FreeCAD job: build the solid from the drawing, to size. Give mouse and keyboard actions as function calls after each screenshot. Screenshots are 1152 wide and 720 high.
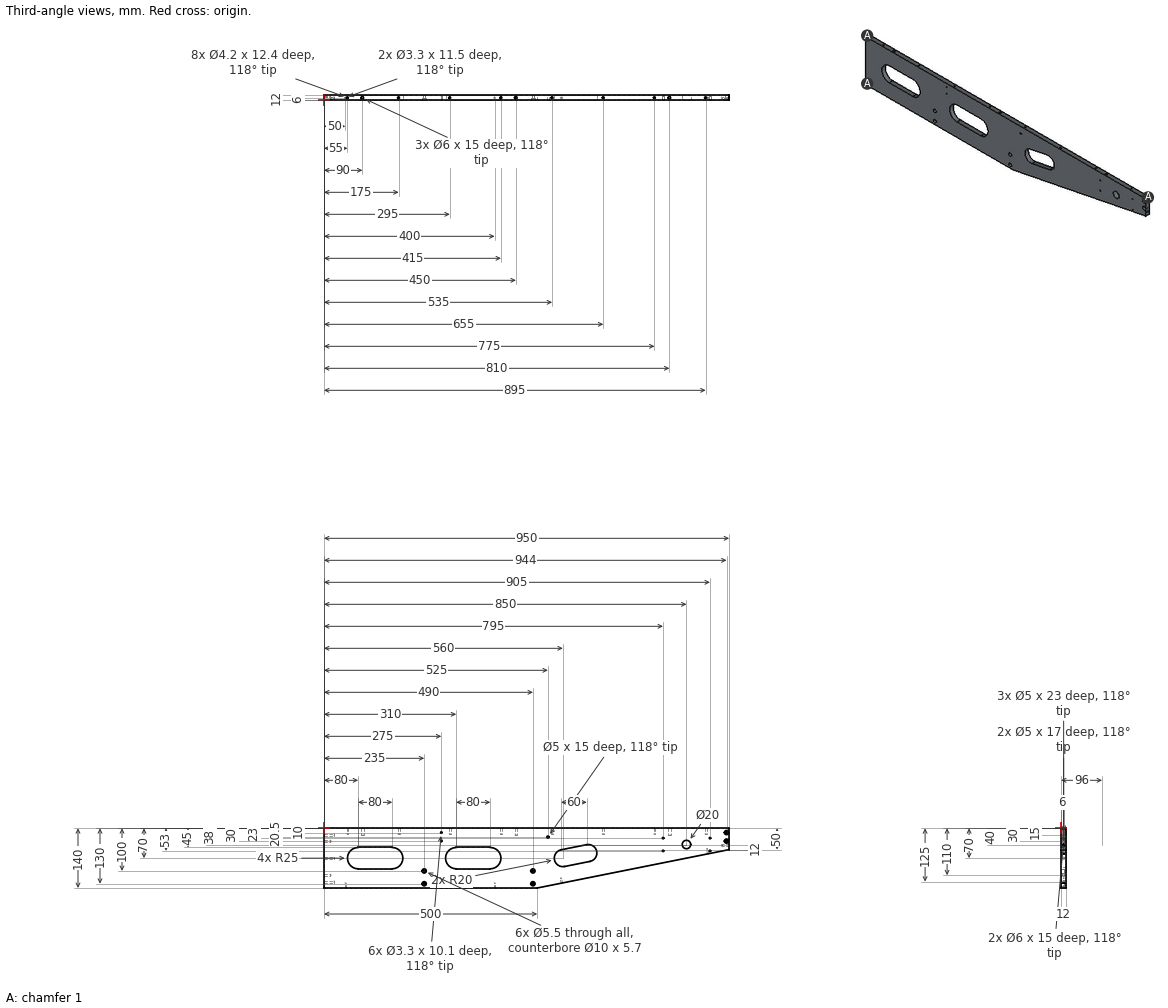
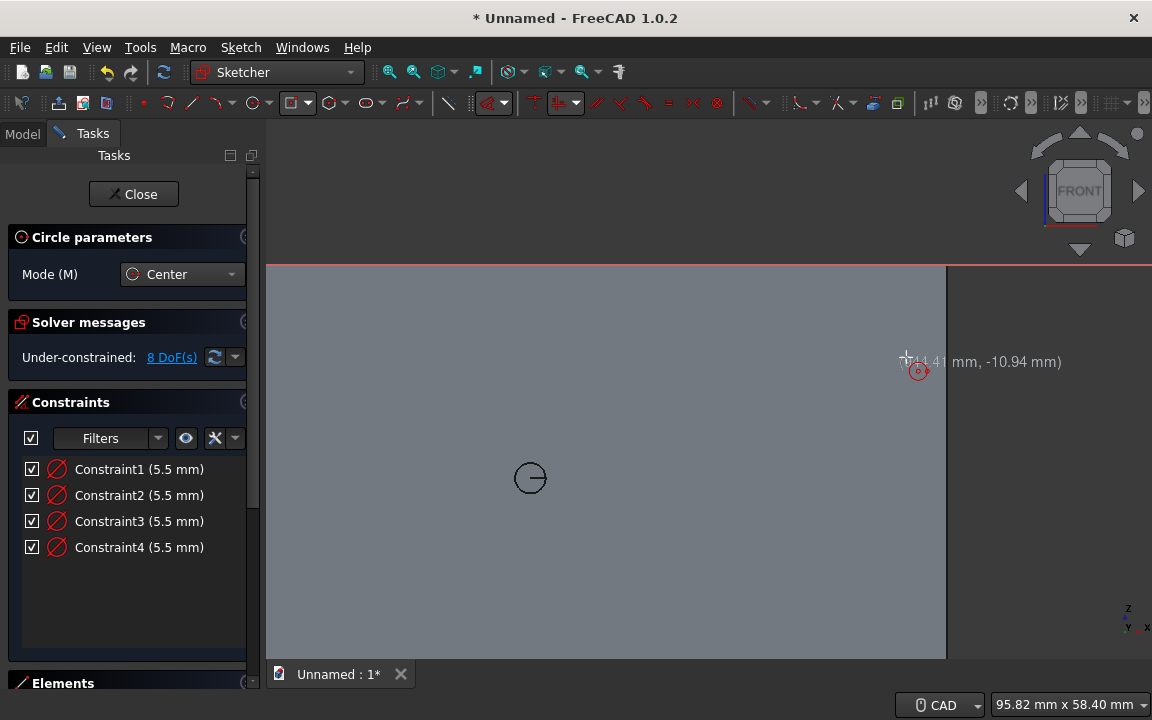
scroll(906, 357, down, 14)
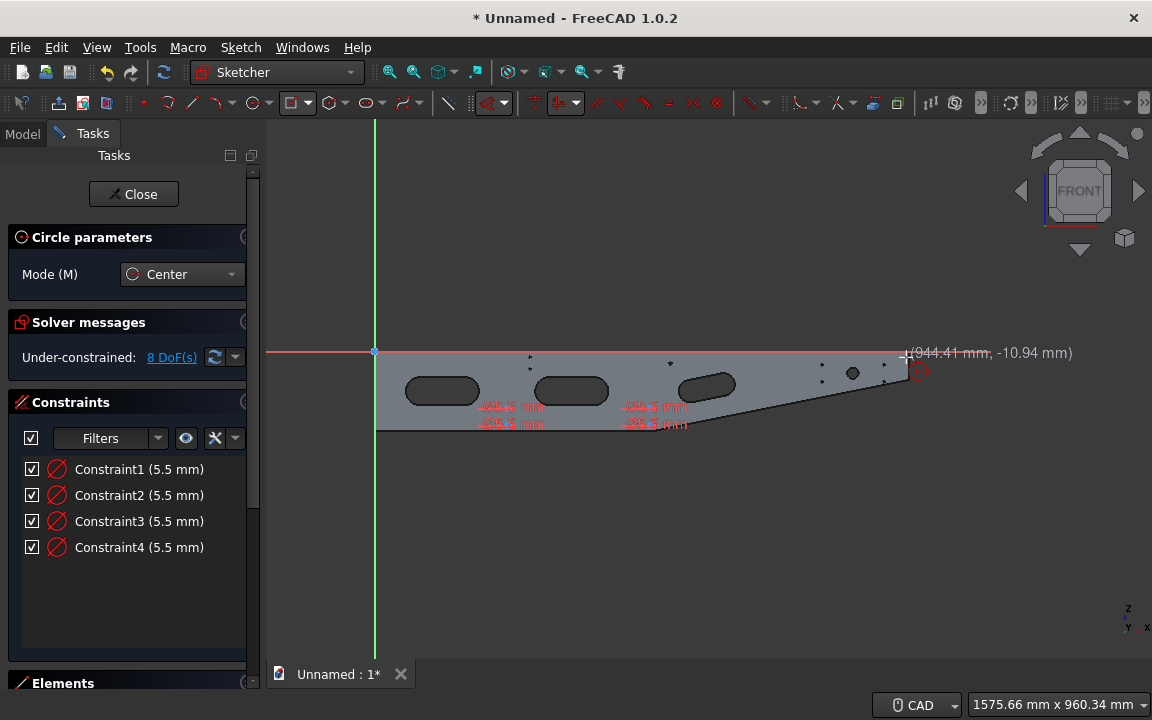
scroll(906, 357, up, 6)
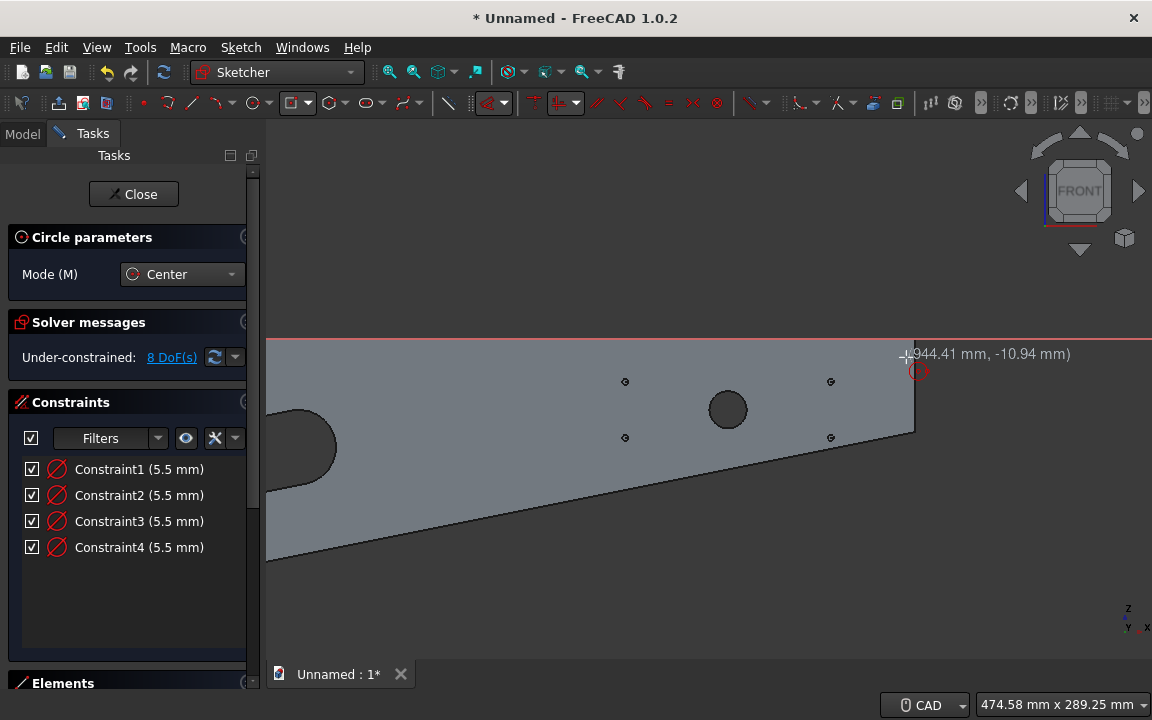
click(904, 358)
move(907, 354)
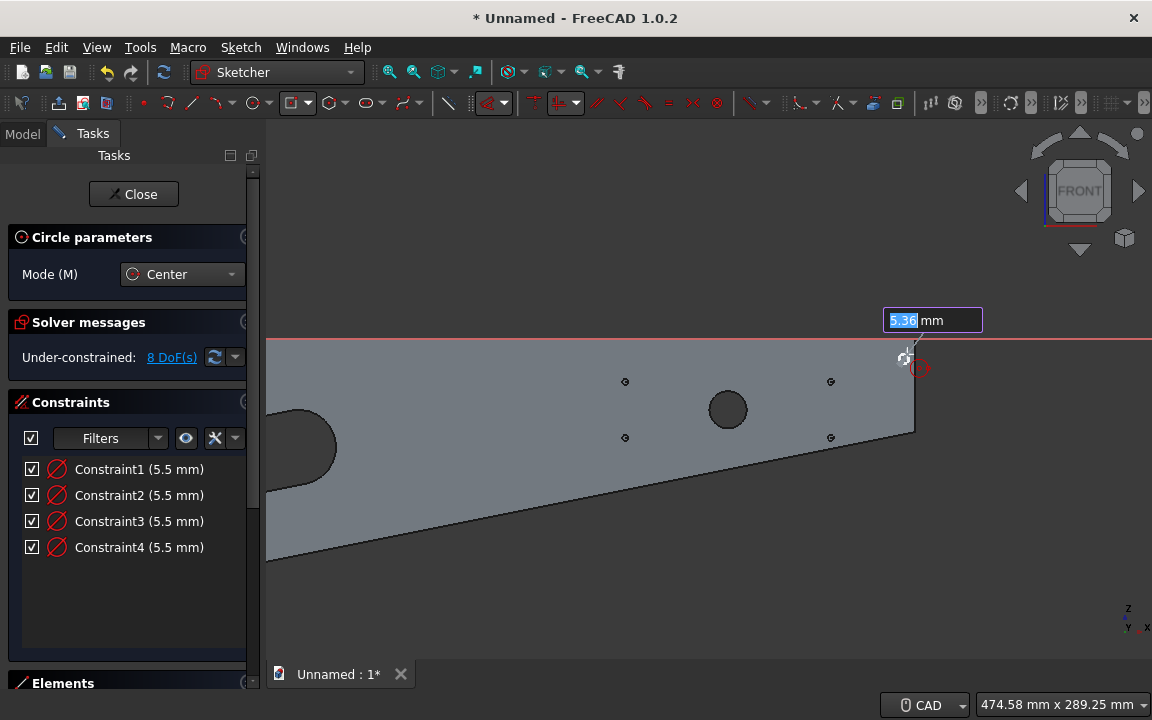
text(5.5)
key(Return)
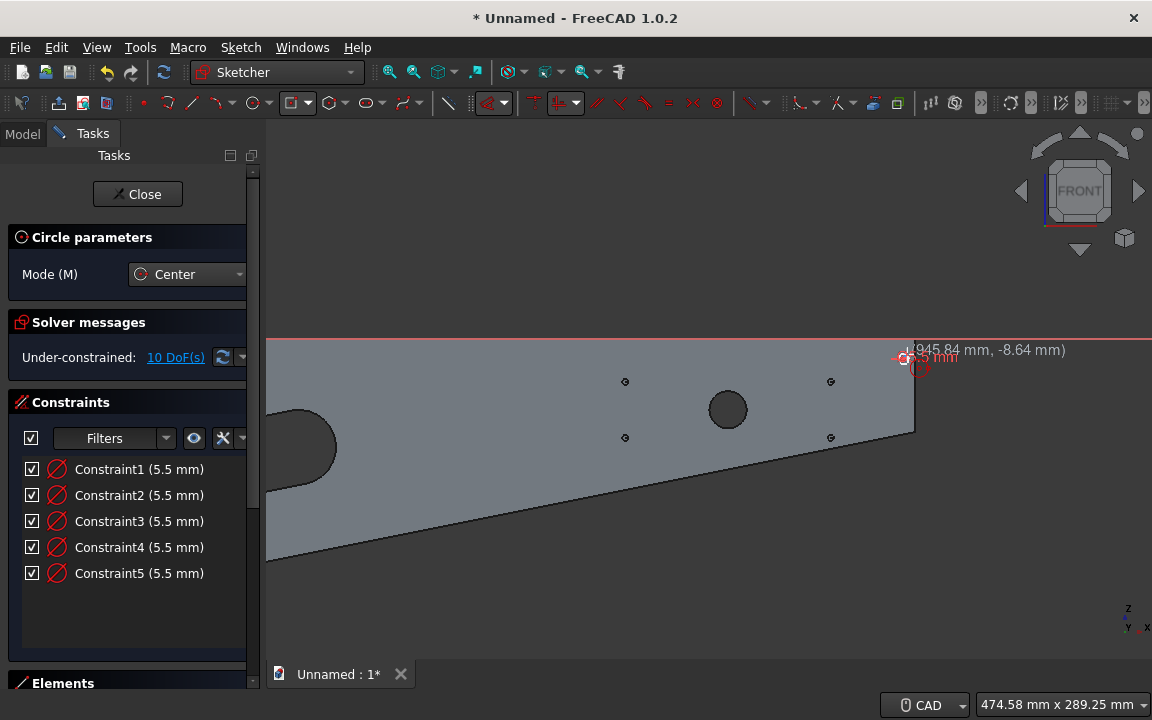
scroll(904, 395, up, 8)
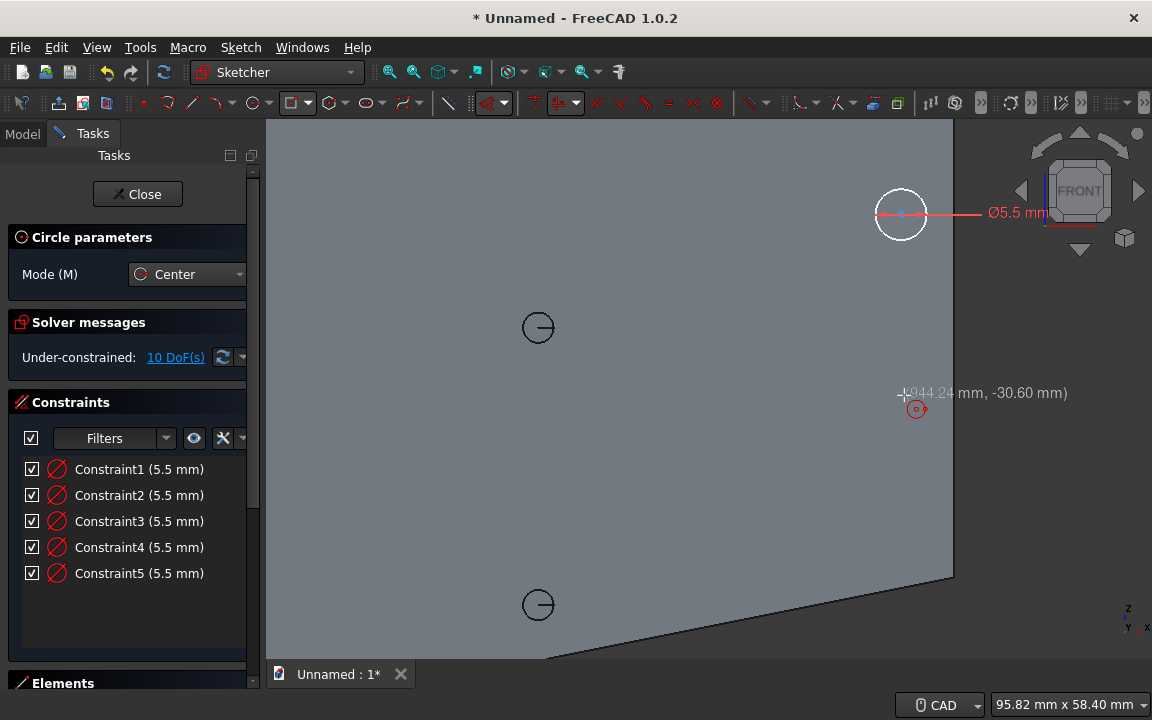
scroll(906, 367, down, 14)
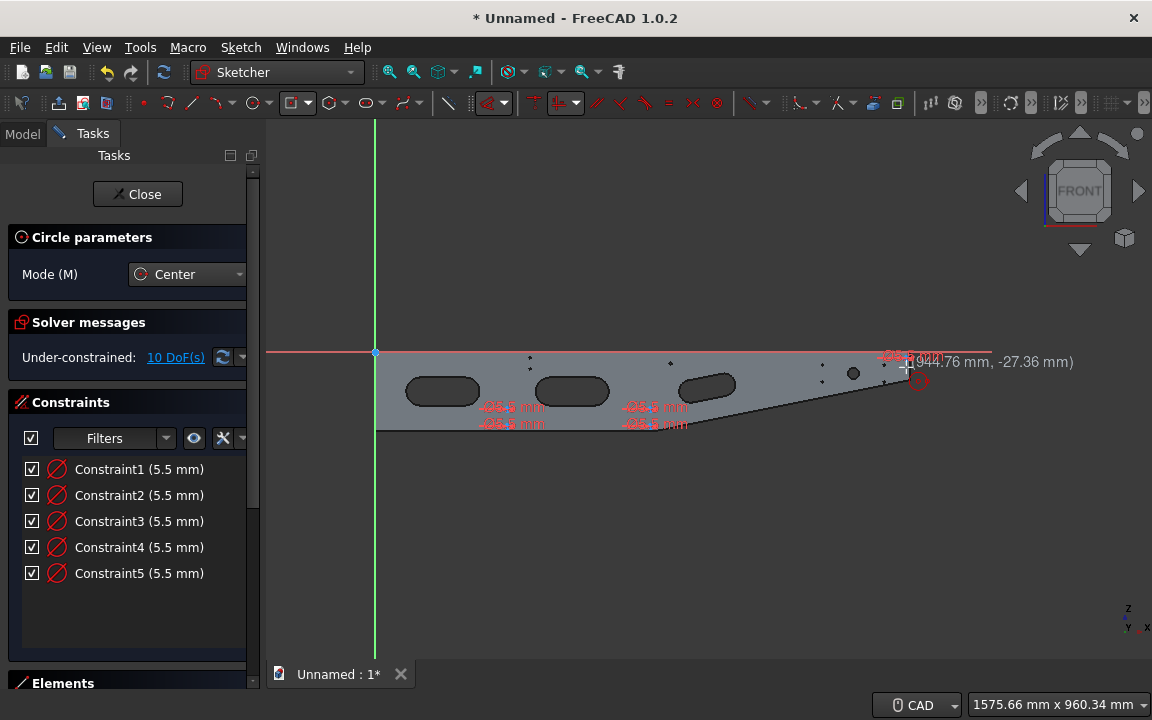
scroll(906, 369, up, 3)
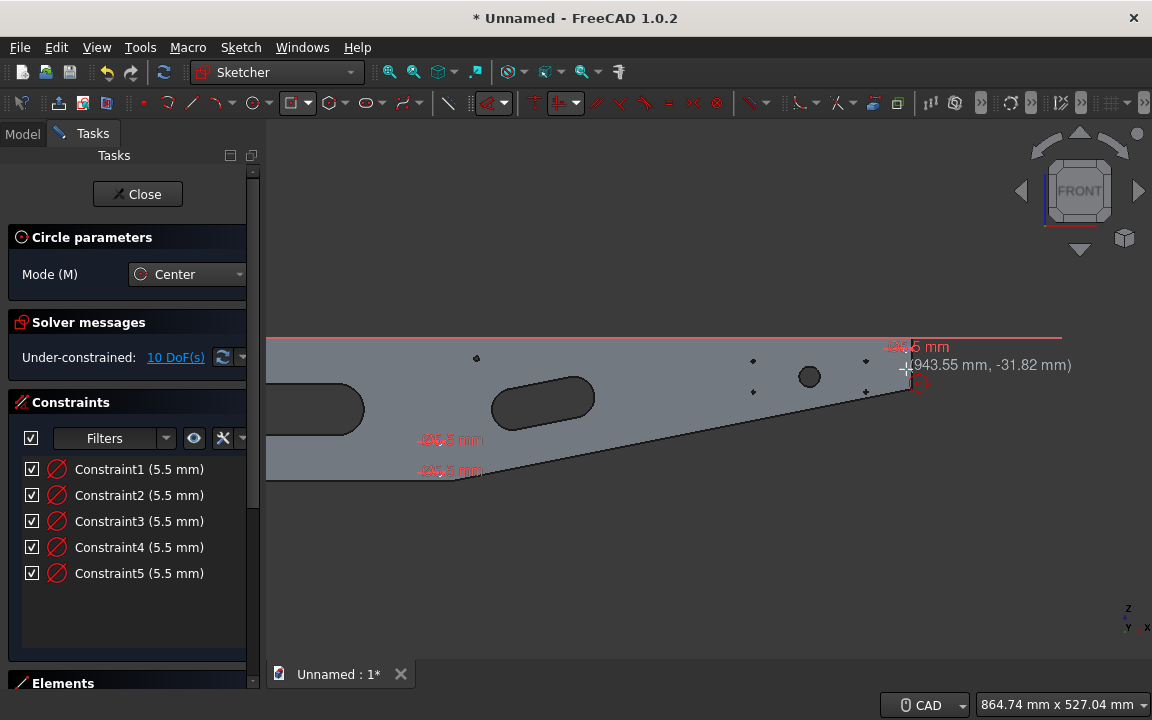
click(906, 369)
move(908, 367)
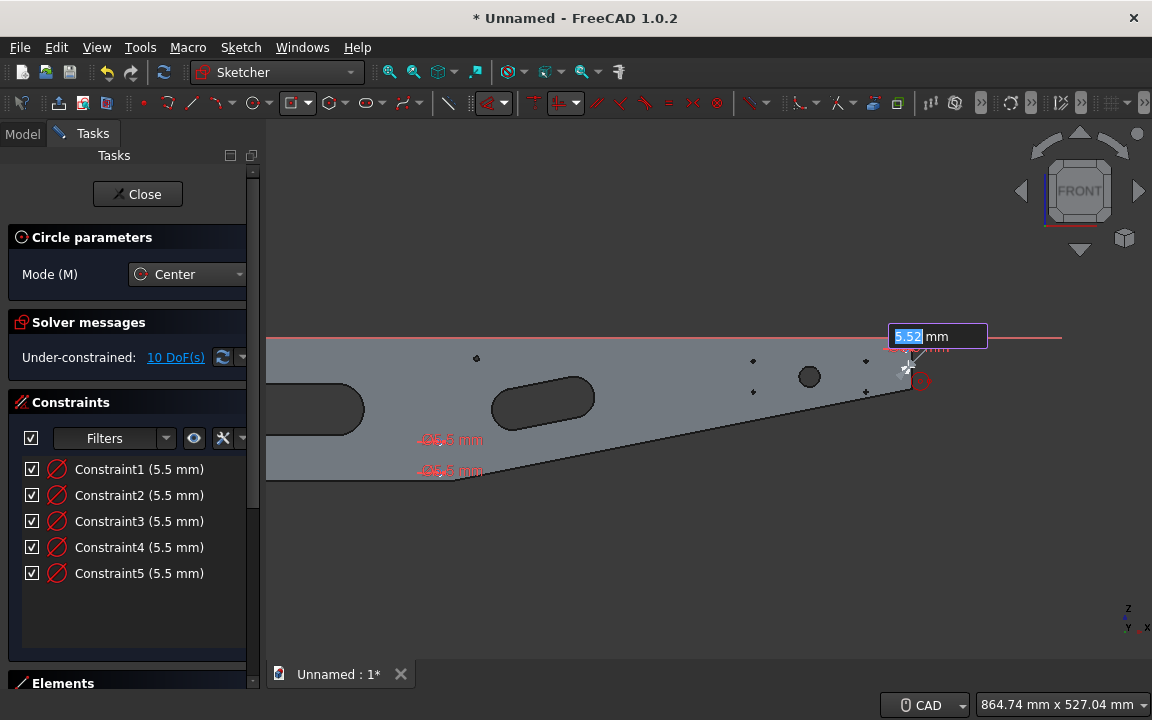
text(5.5)
key(Return)
key(Escape)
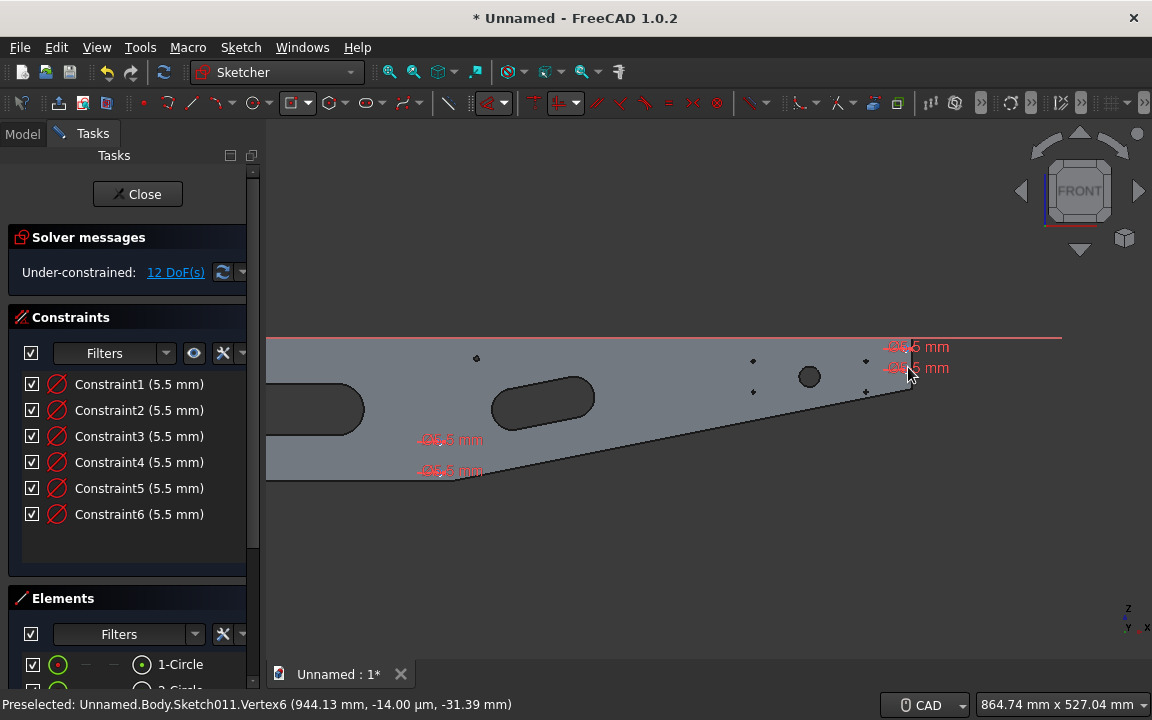
scroll(904, 369, down, 3)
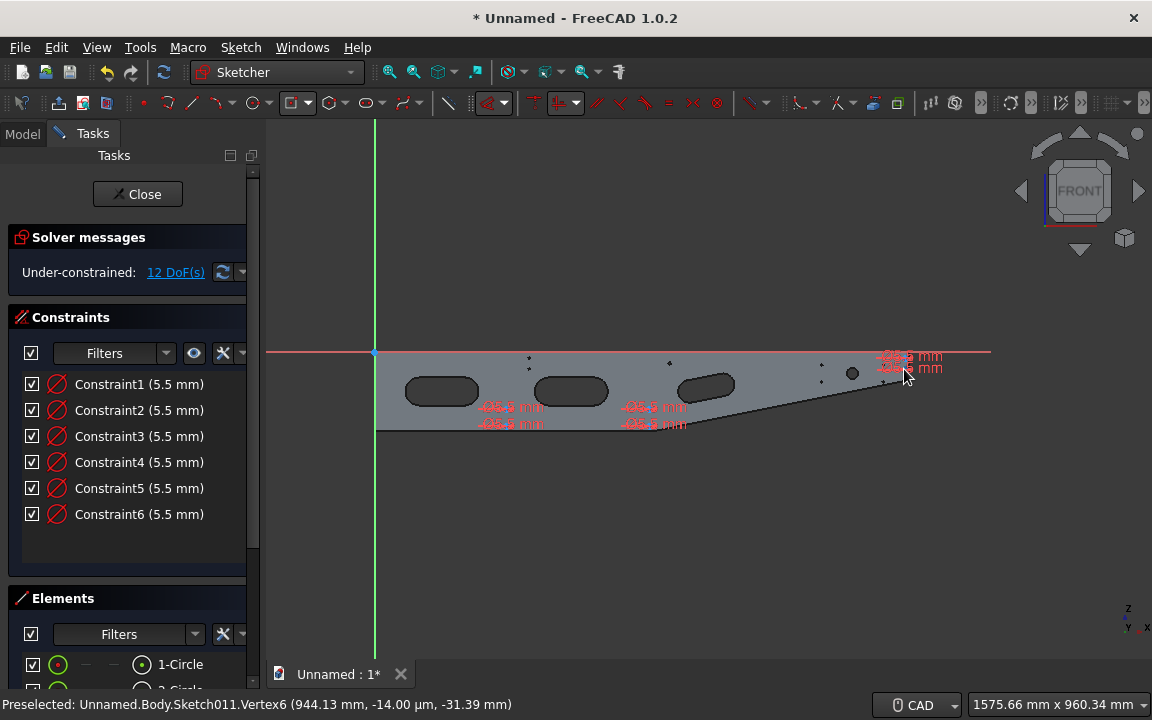
click(507, 409)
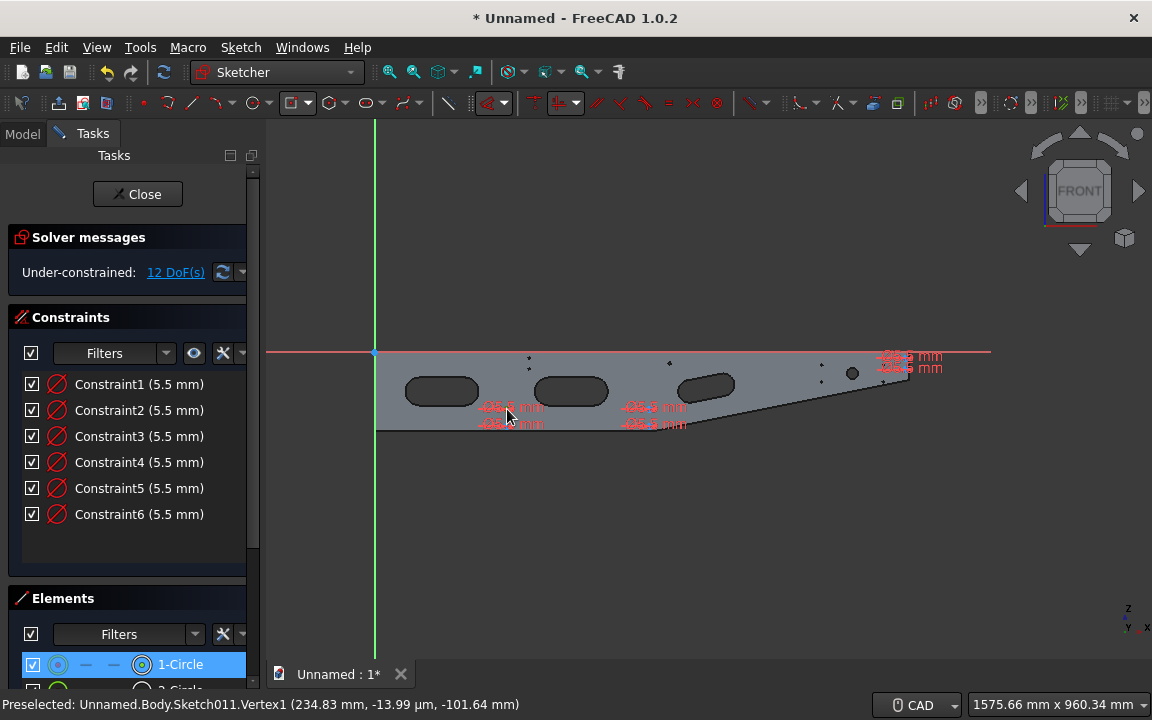
click(507, 426)